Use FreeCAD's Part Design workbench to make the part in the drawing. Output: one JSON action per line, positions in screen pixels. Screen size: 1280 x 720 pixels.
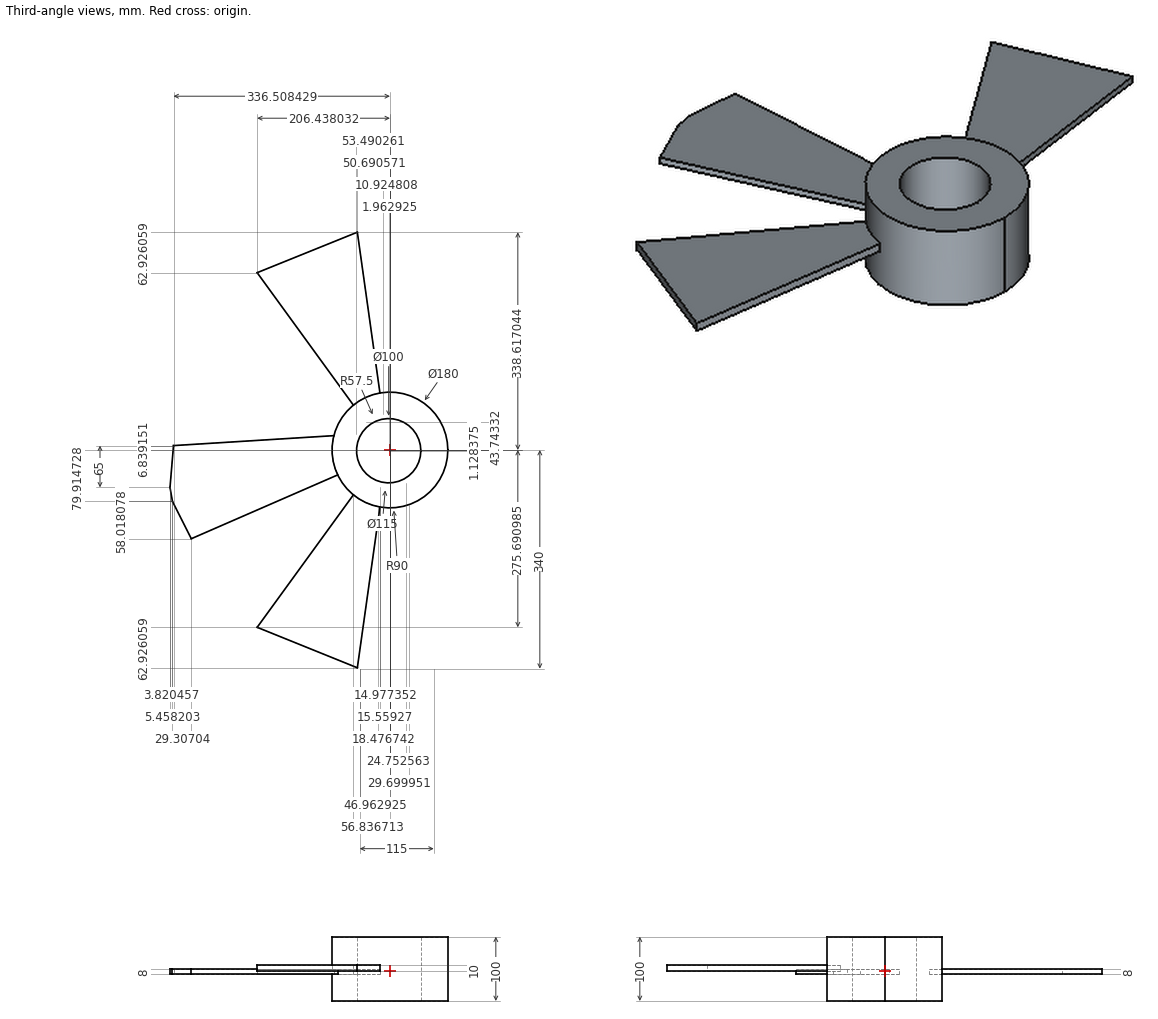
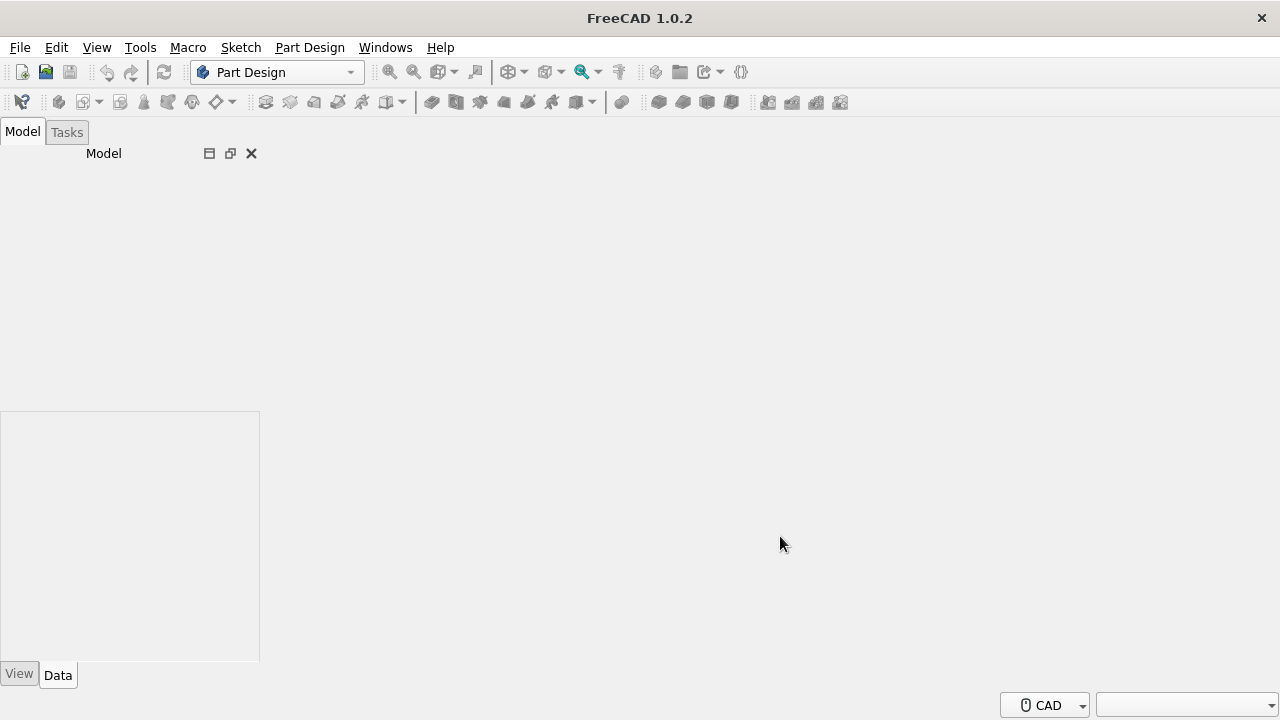
{"action": "left_click", "coordinate": [22, 72]}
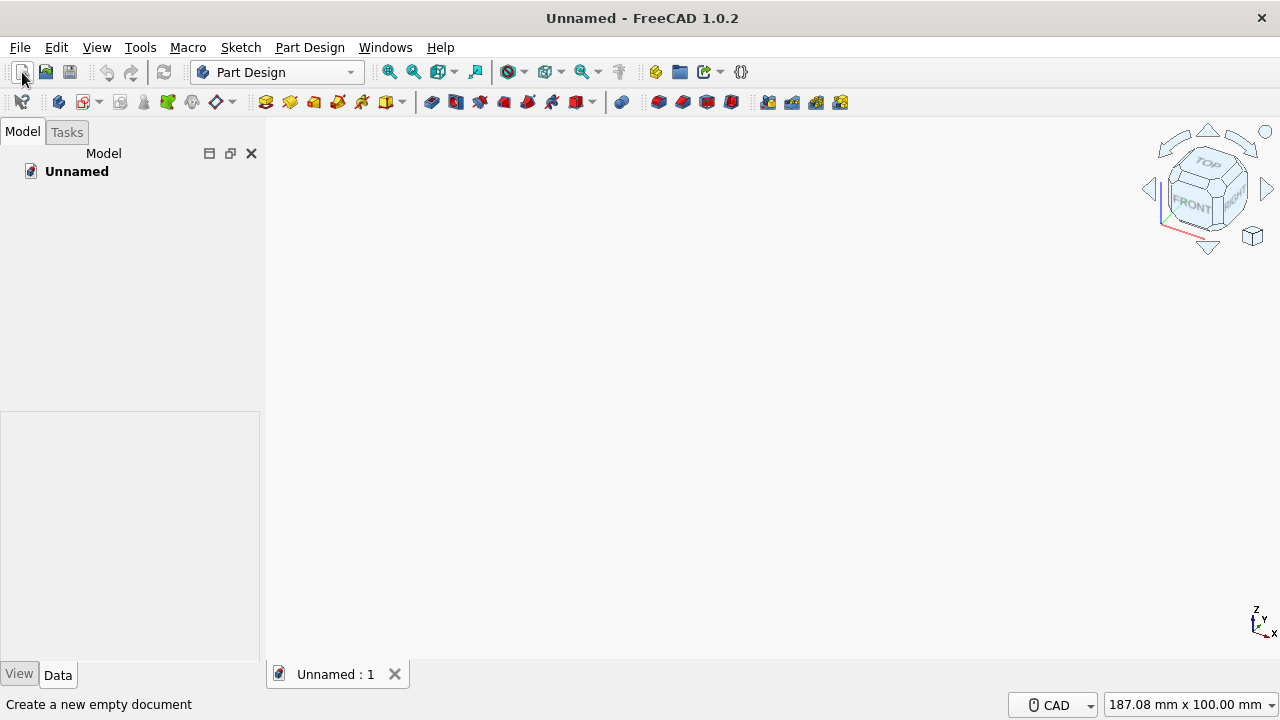
{"action": "left_click", "coordinate": [84, 102]}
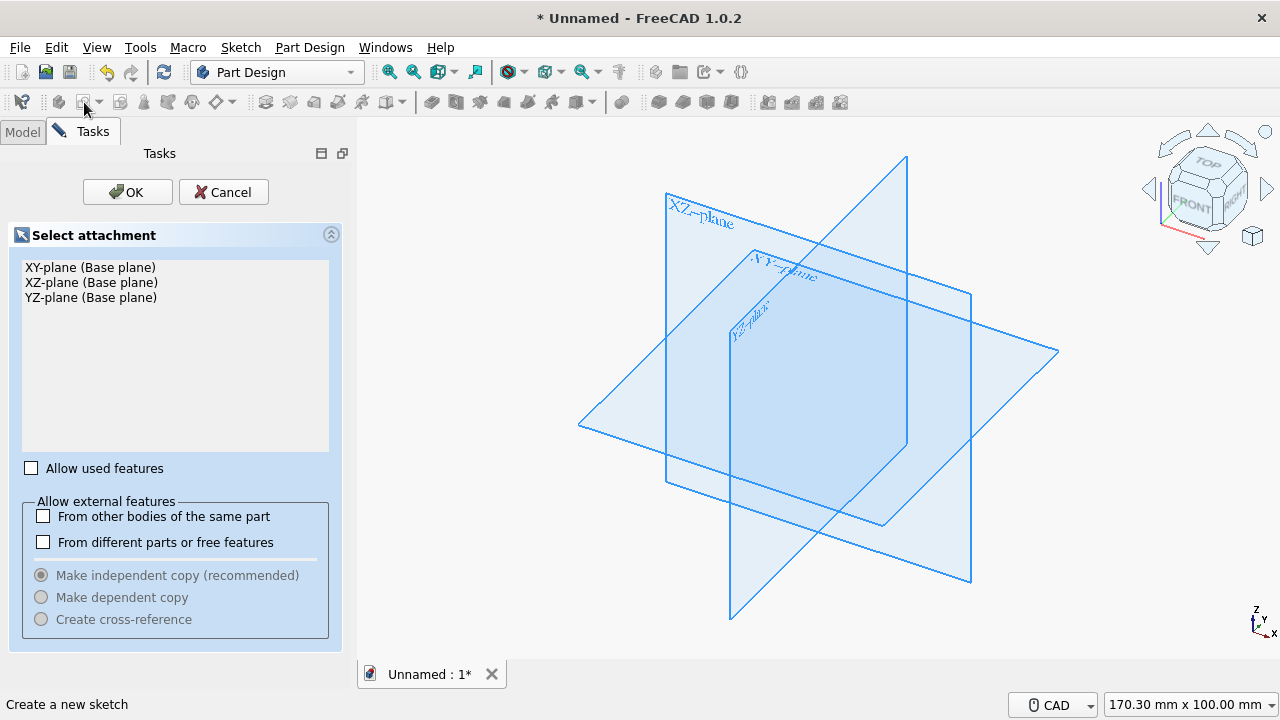
{"action": "left_click", "coordinate": [82, 268]}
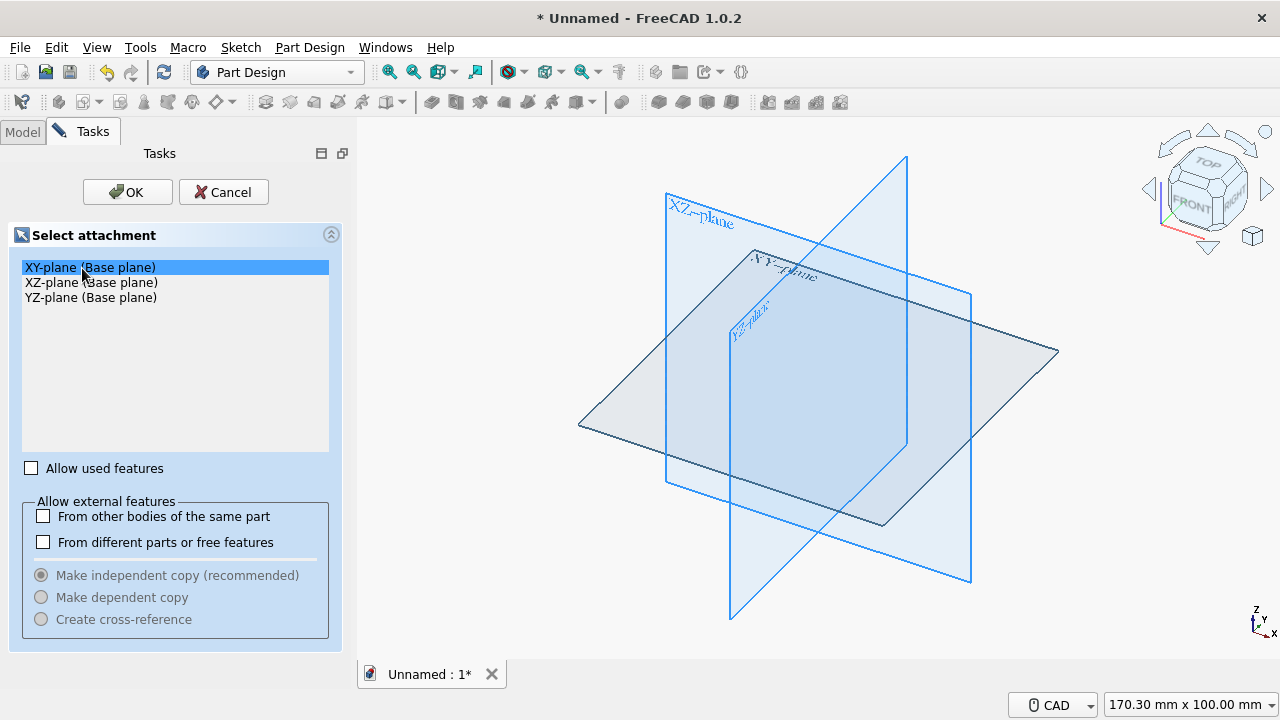
{"action": "left_click", "coordinate": [128, 192]}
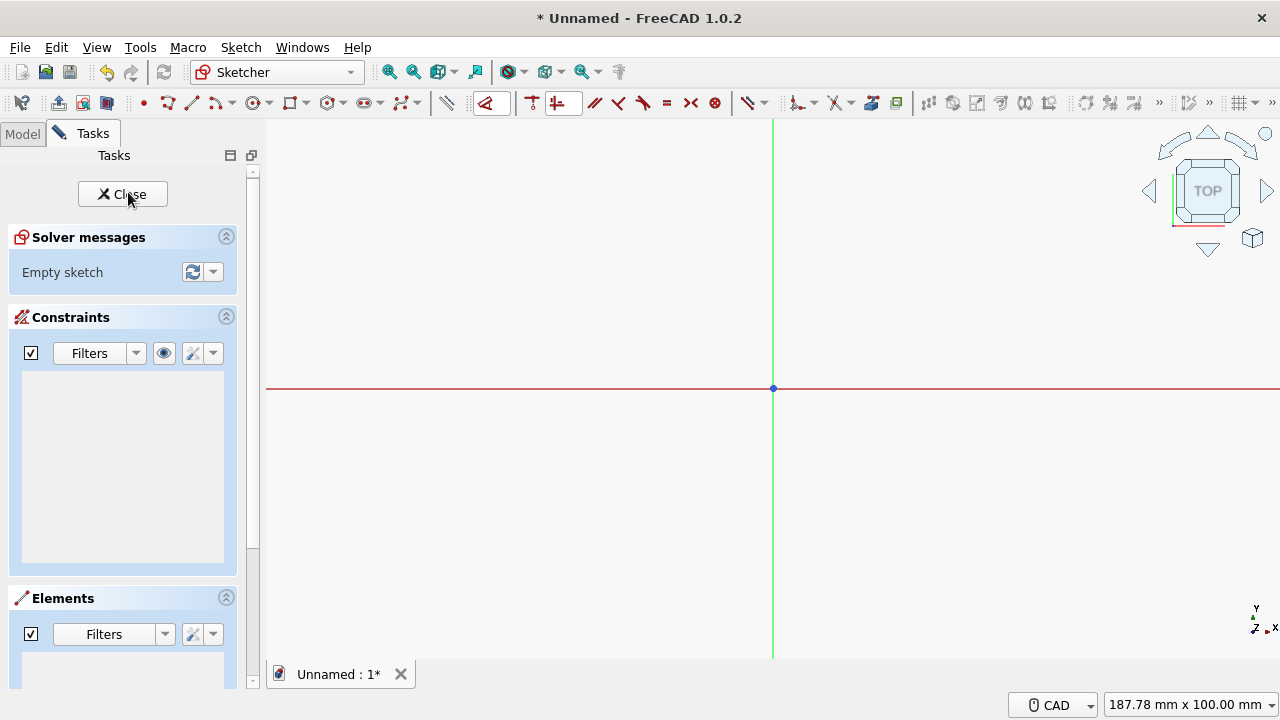
{"action": "scroll", "coordinate": [828, 620], "scroll_direction": "down", "scroll_amount": 8}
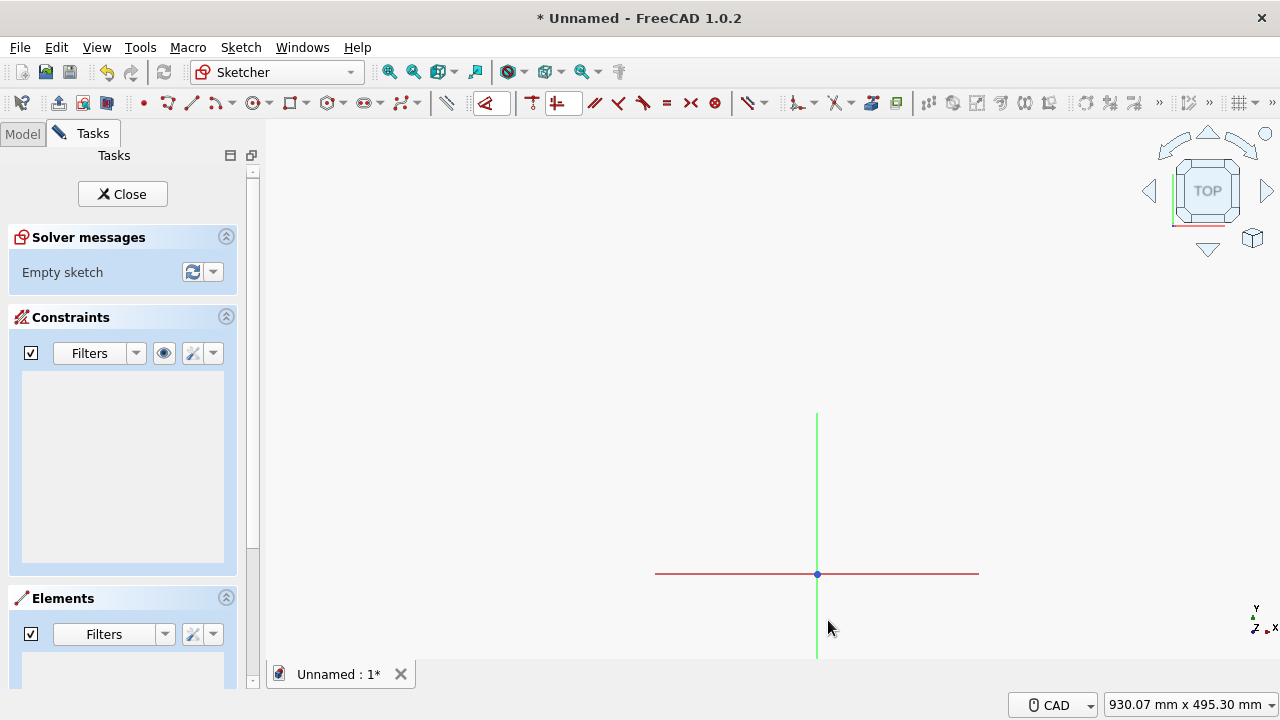
{"action": "left_click", "coordinate": [168, 104]}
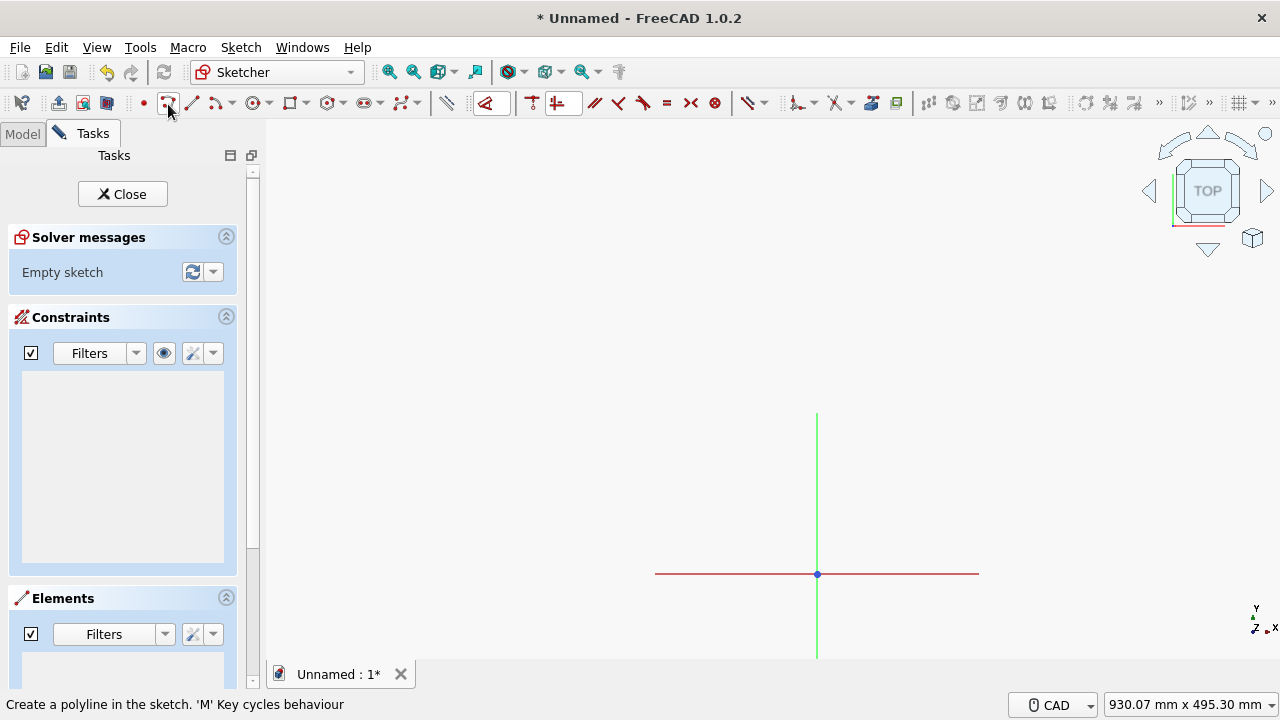
{"action": "scroll", "coordinate": [805, 513], "scroll_direction": "up", "scroll_amount": 2}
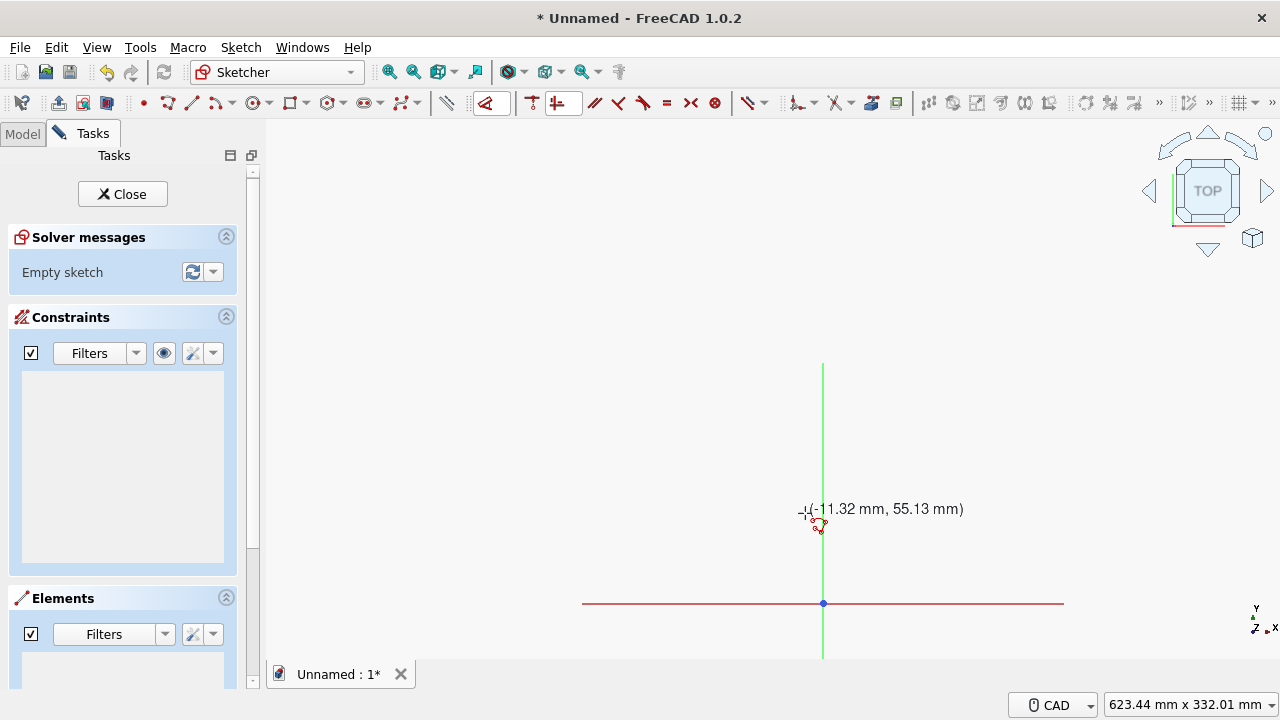
{"action": "left_click", "coordinate": [805, 513]}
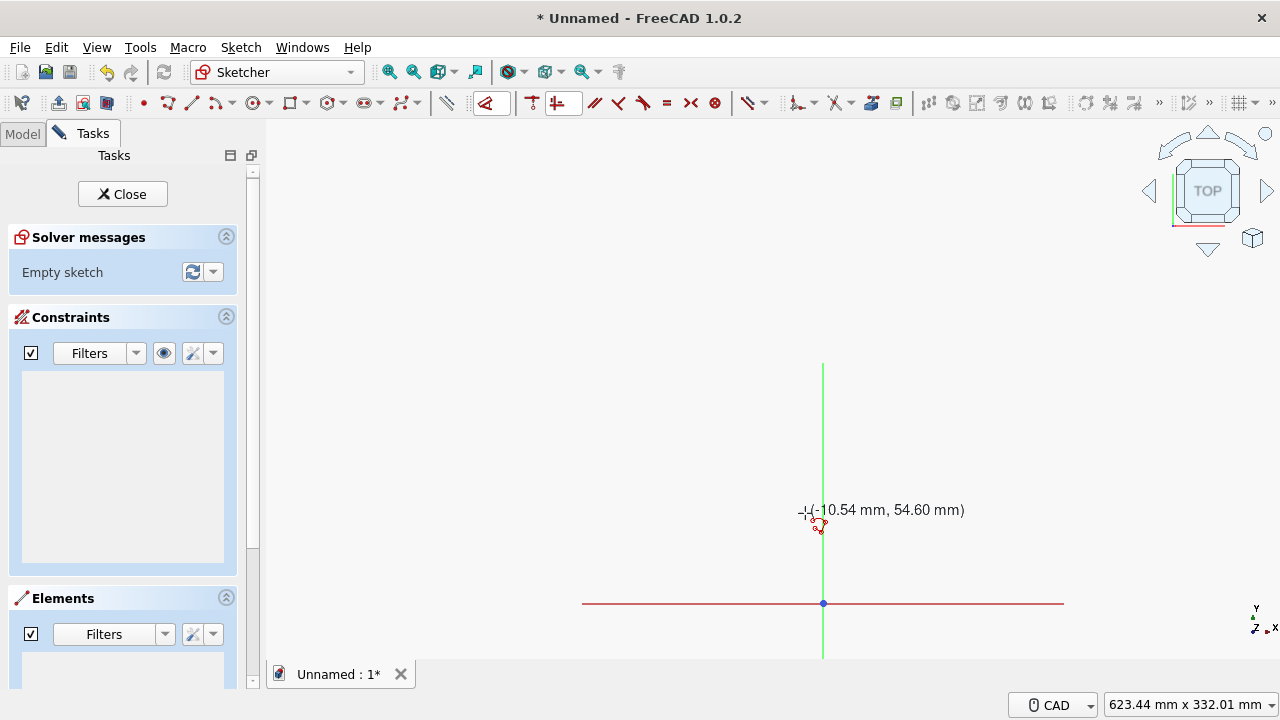
{"action": "scroll", "coordinate": [805, 512], "scroll_direction": "down", "scroll_amount": 2}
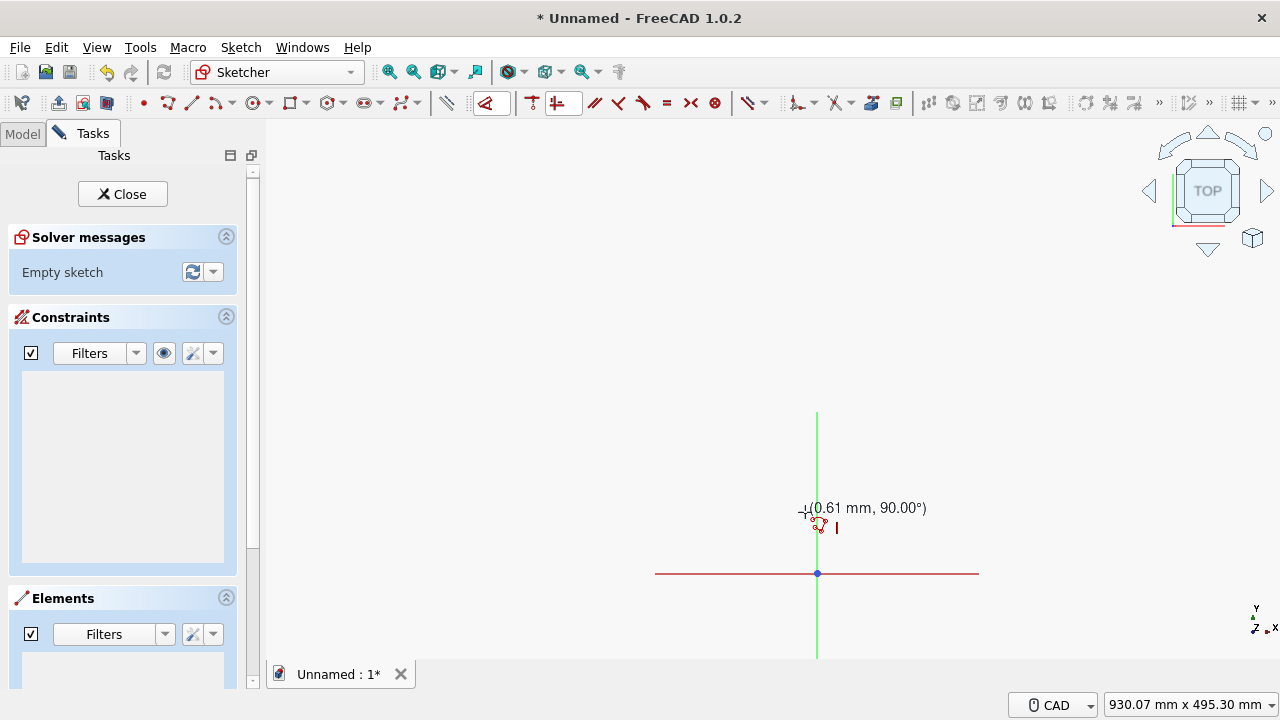
{"action": "left_click", "coordinate": [762, 205]}
{"action": "left_click", "coordinate": [592, 273]}
{"action": "left_click", "coordinate": [776, 526]}
{"action": "right_click", "coordinate": [776, 526]}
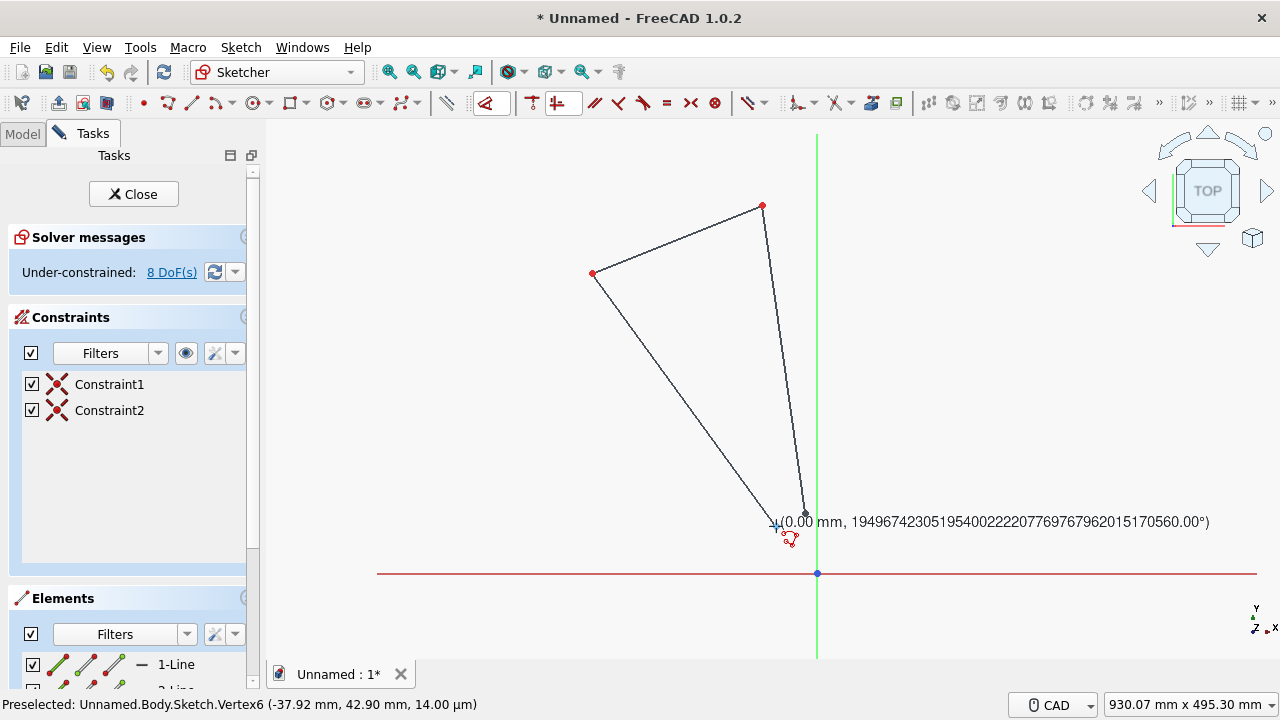
{"action": "left_click", "coordinate": [234, 104]}